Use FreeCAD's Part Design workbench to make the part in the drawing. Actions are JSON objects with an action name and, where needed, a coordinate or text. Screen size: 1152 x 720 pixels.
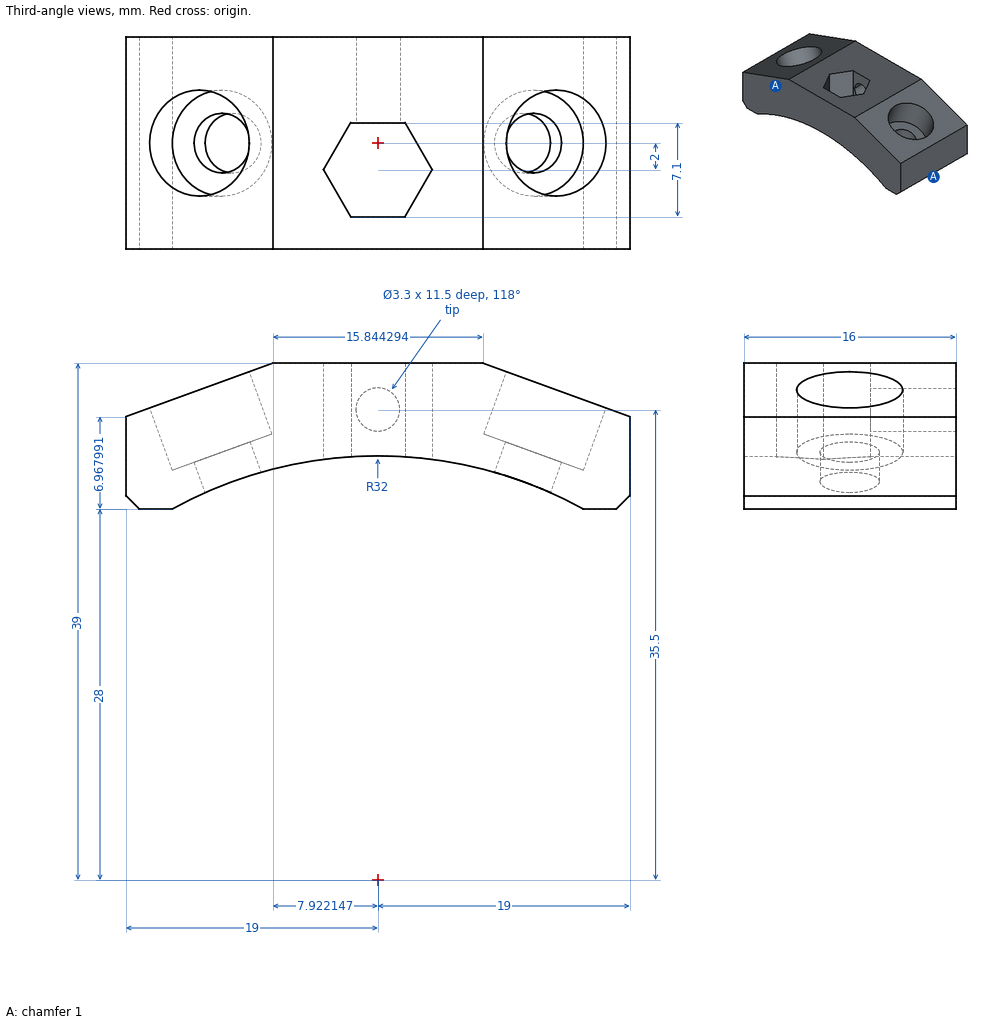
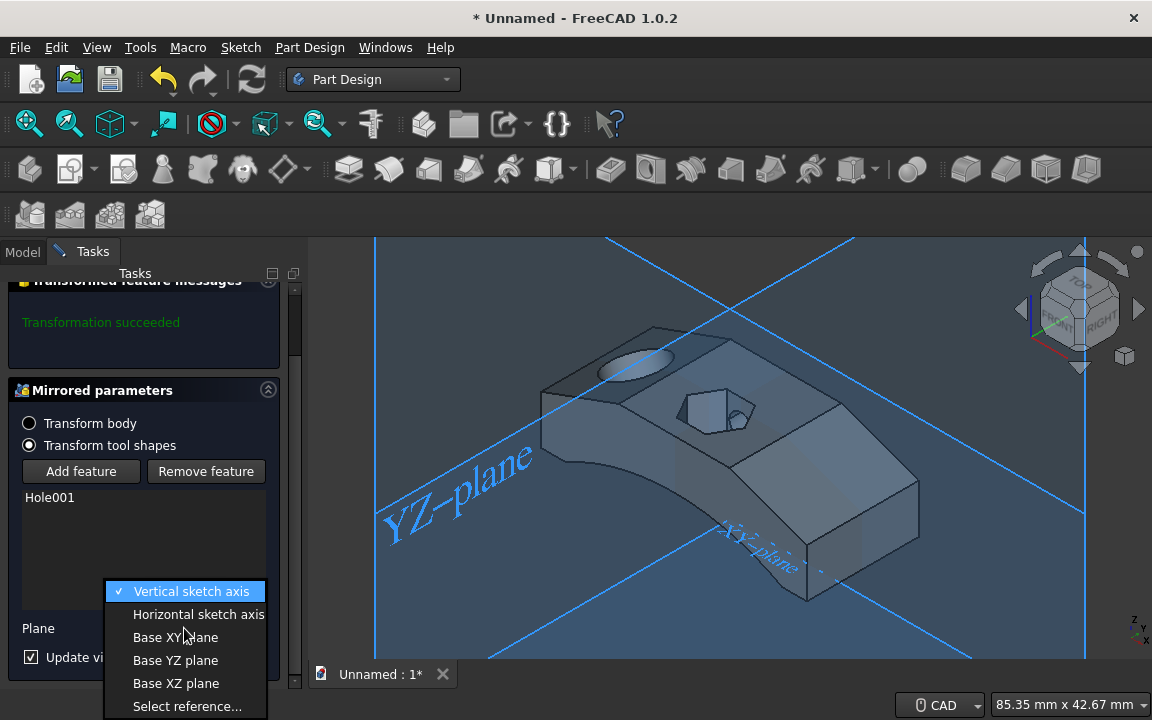
{"action": "left_click", "coordinate": [184, 660]}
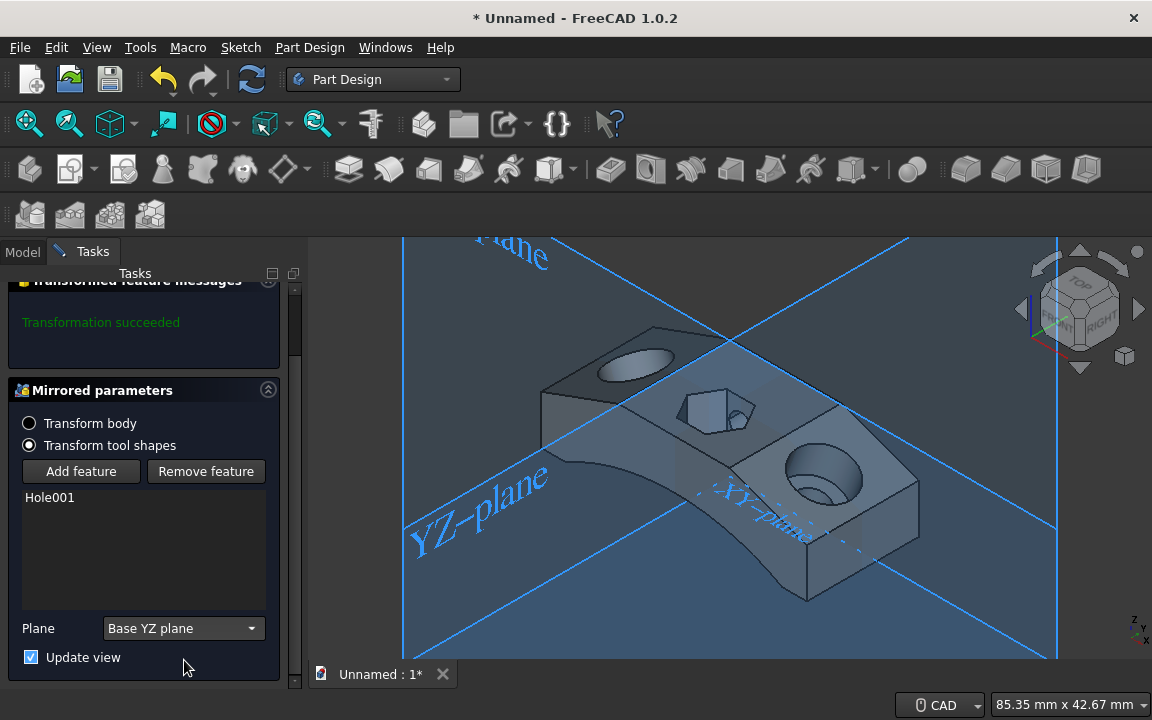
{"action": "scroll", "coordinate": [295, 486], "scroll_direction": "up", "scroll_amount": 2}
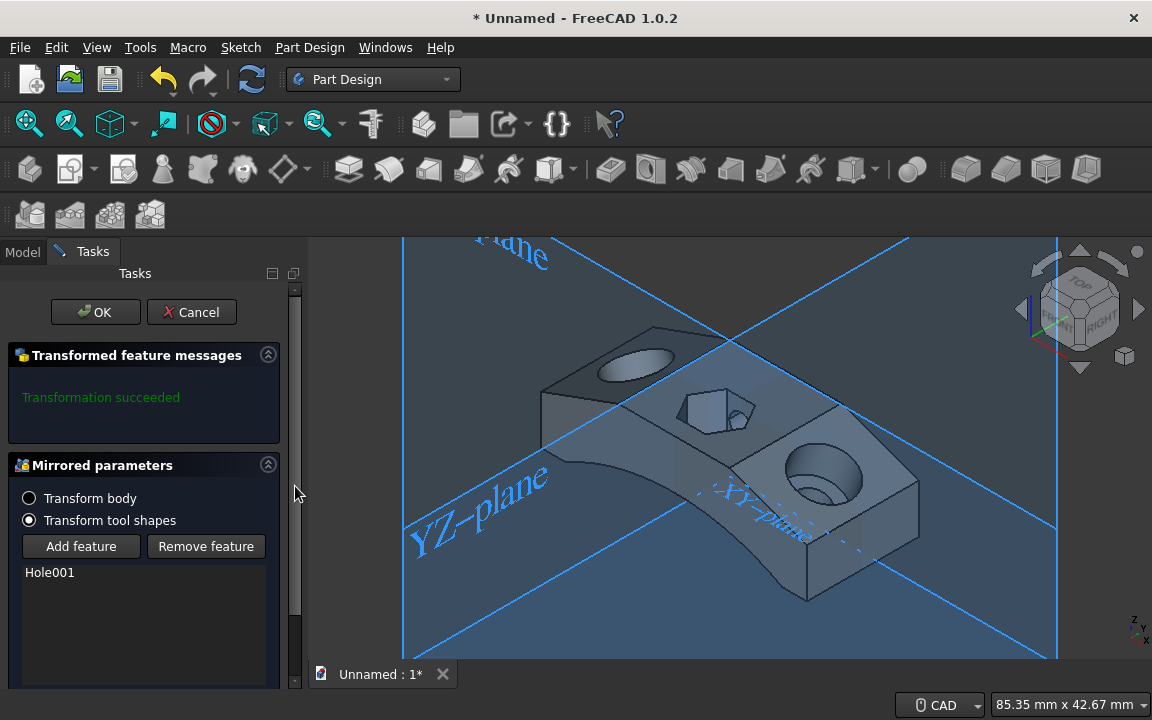
{"action": "left_click", "coordinate": [96, 312]}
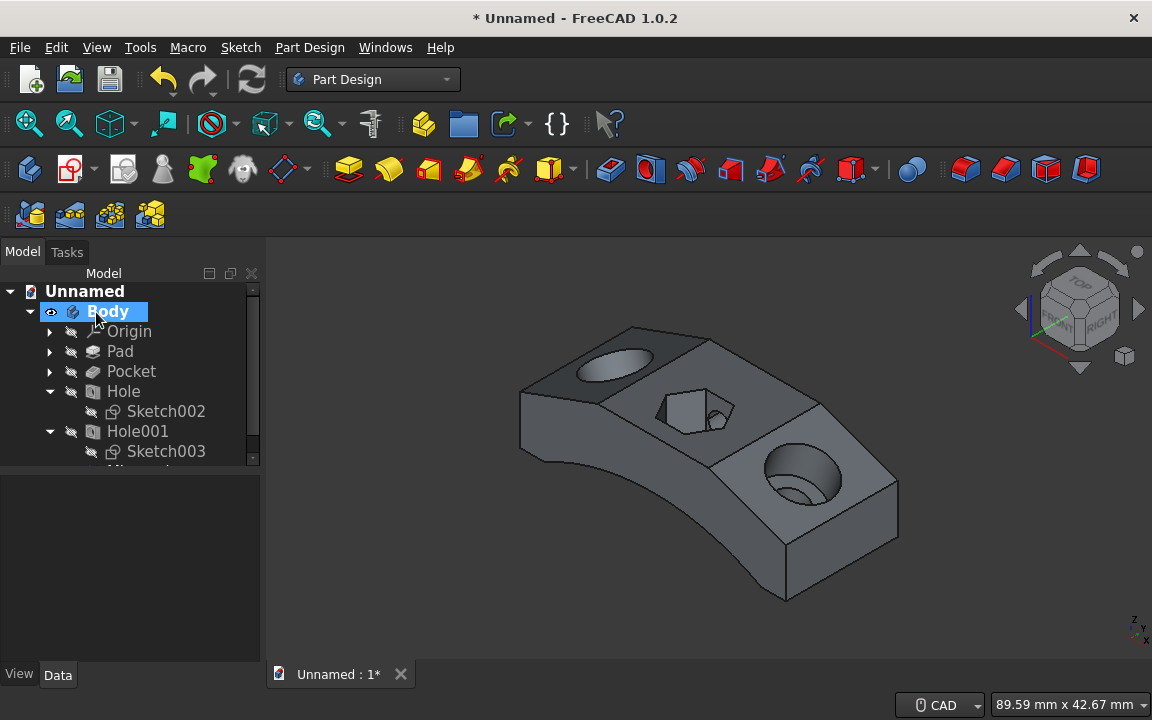
{"action": "key", "text": "2"}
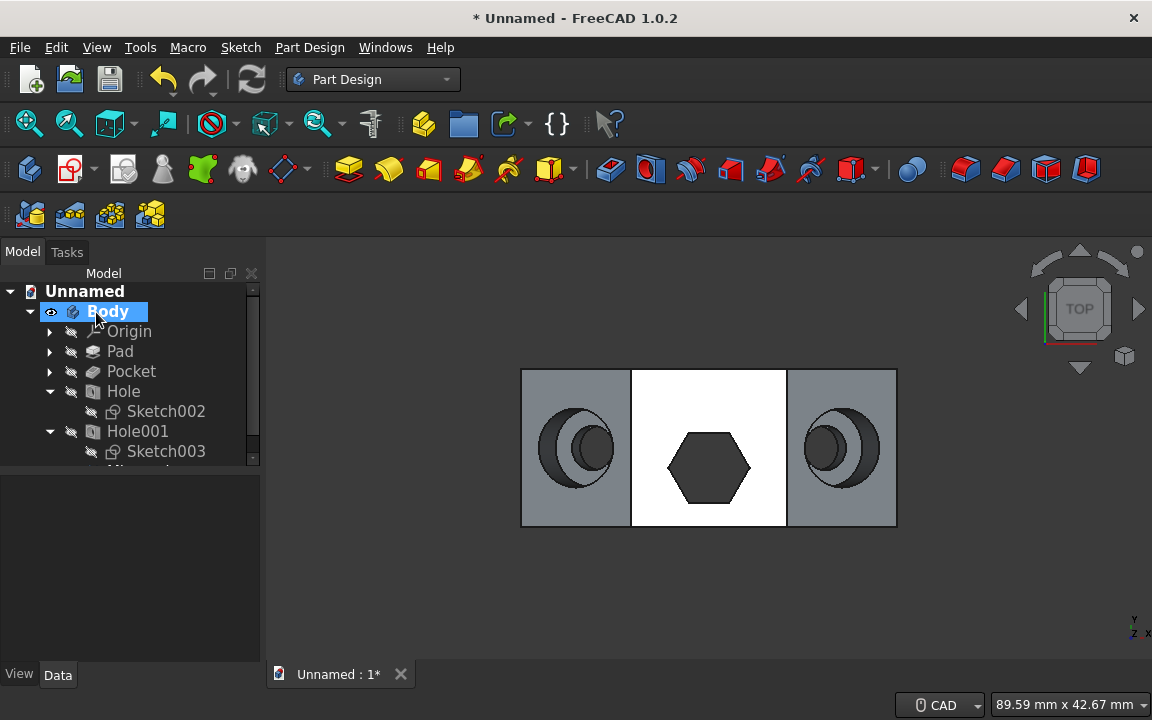
{"action": "key", "text": "v f"}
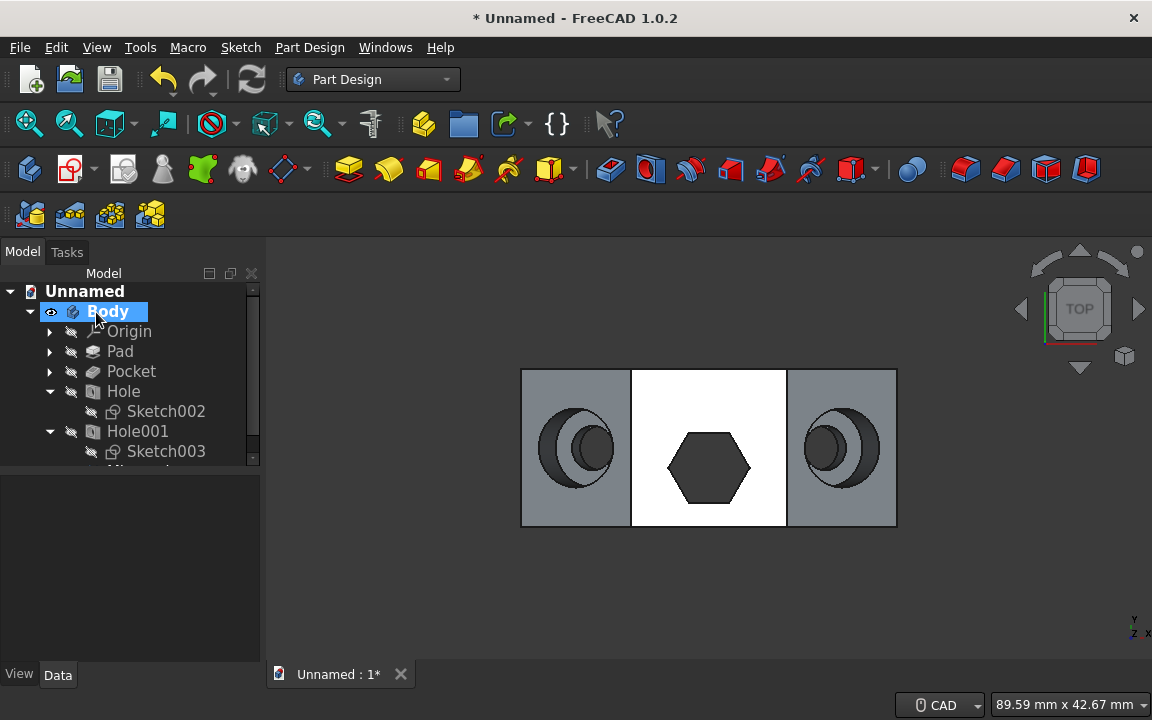
{"action": "key", "text": "0"}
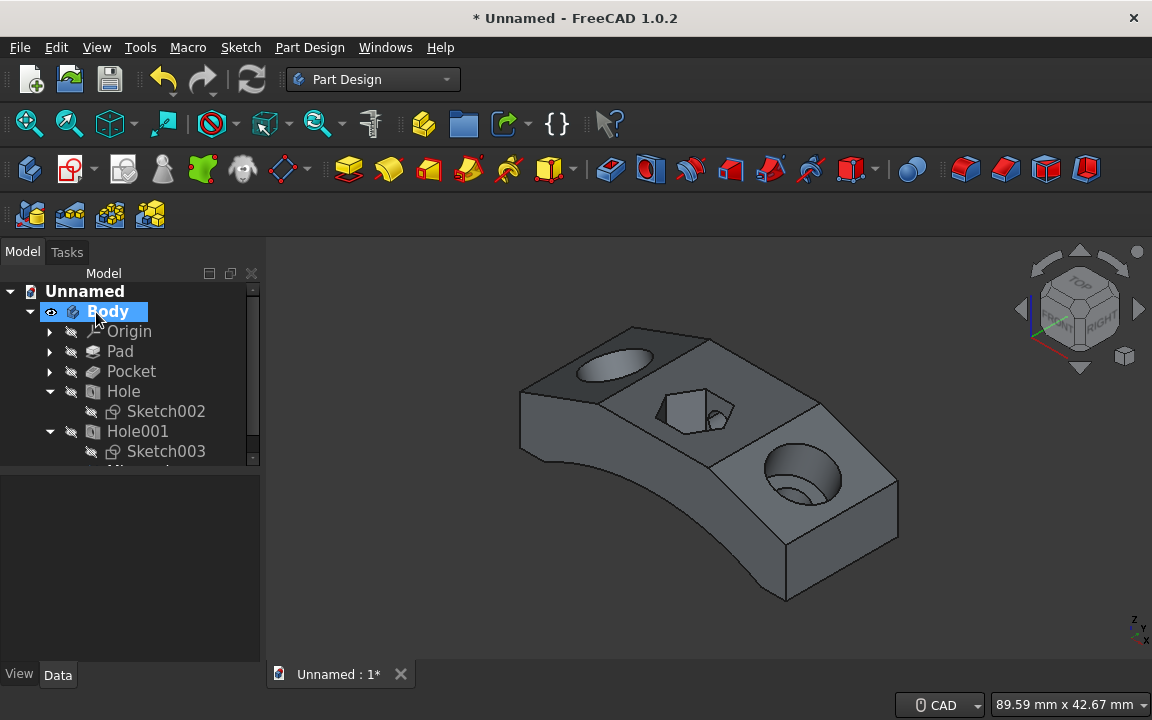
{"action": "key", "text": "1"}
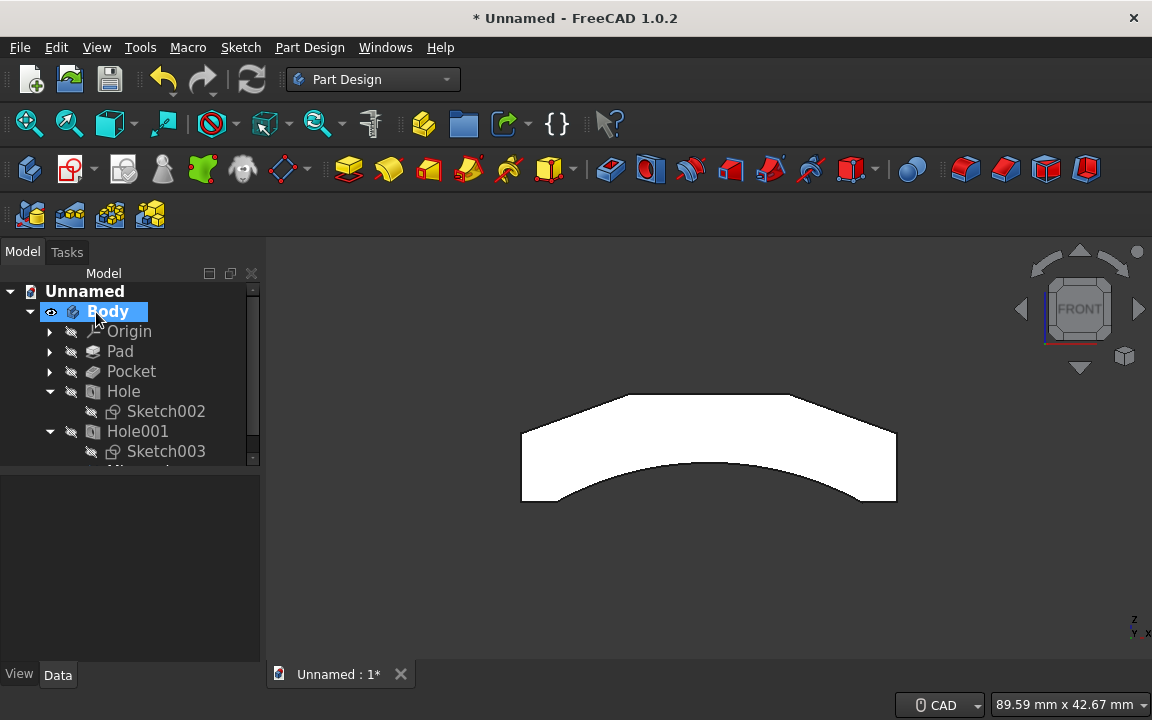
{"action": "key", "text": "v f"}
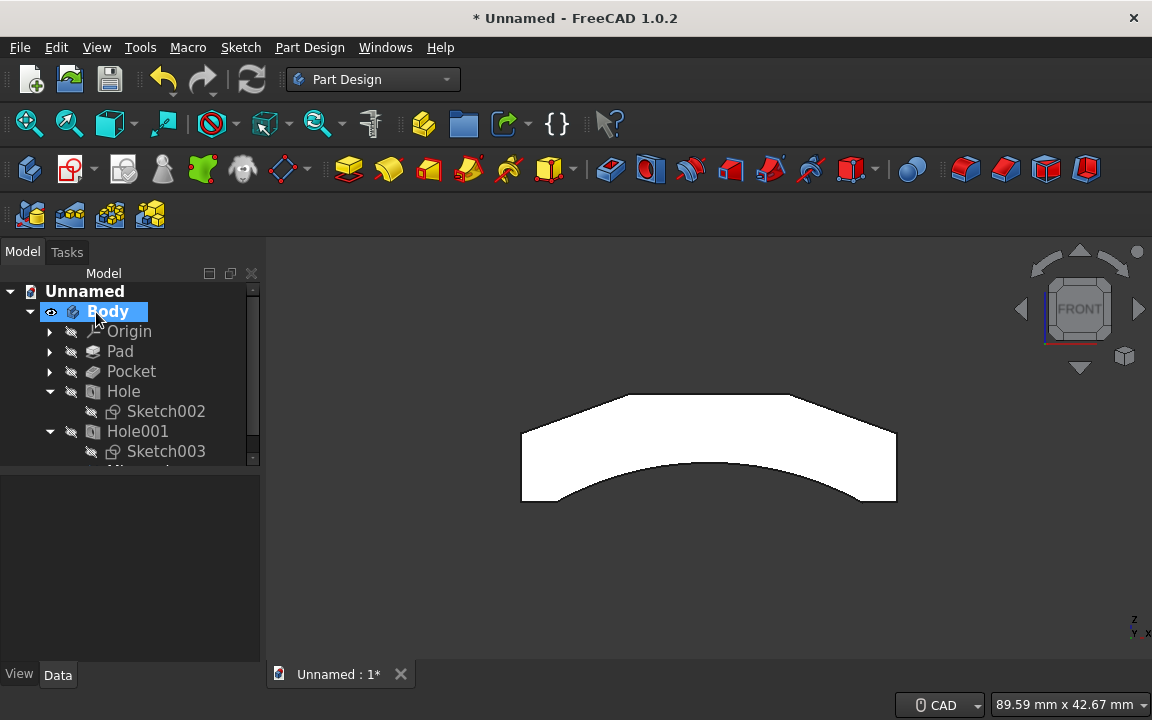
{"action": "key", "text": "3"}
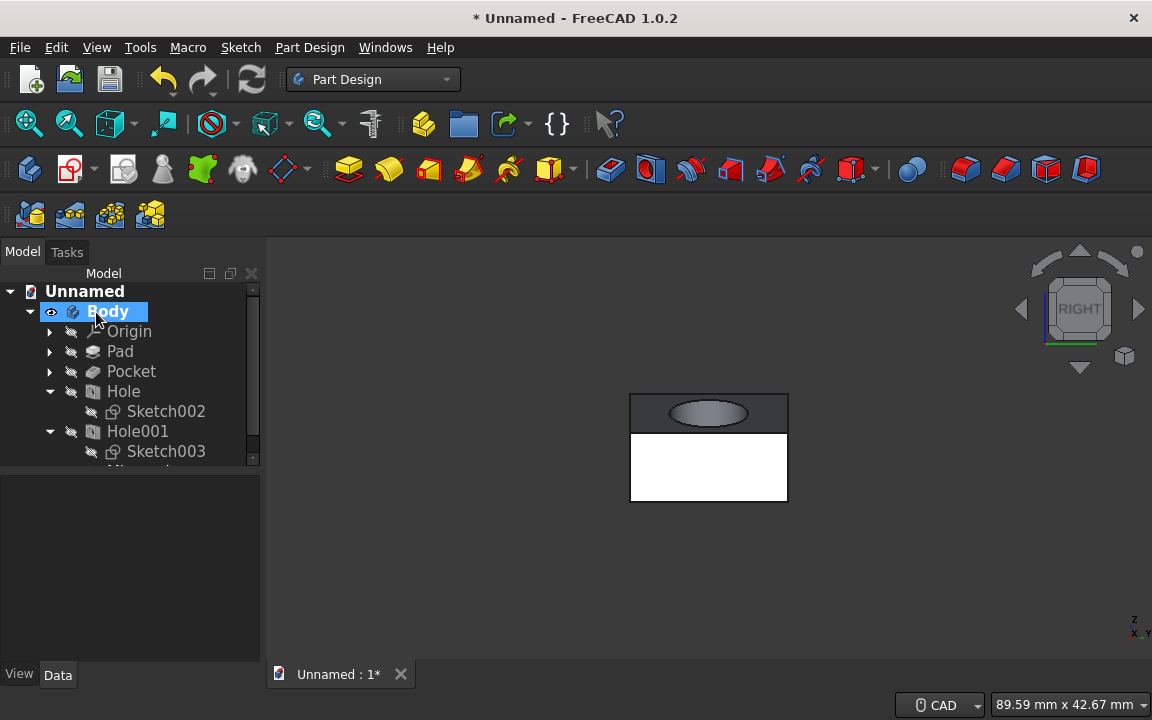
{"action": "key", "text": "v f"}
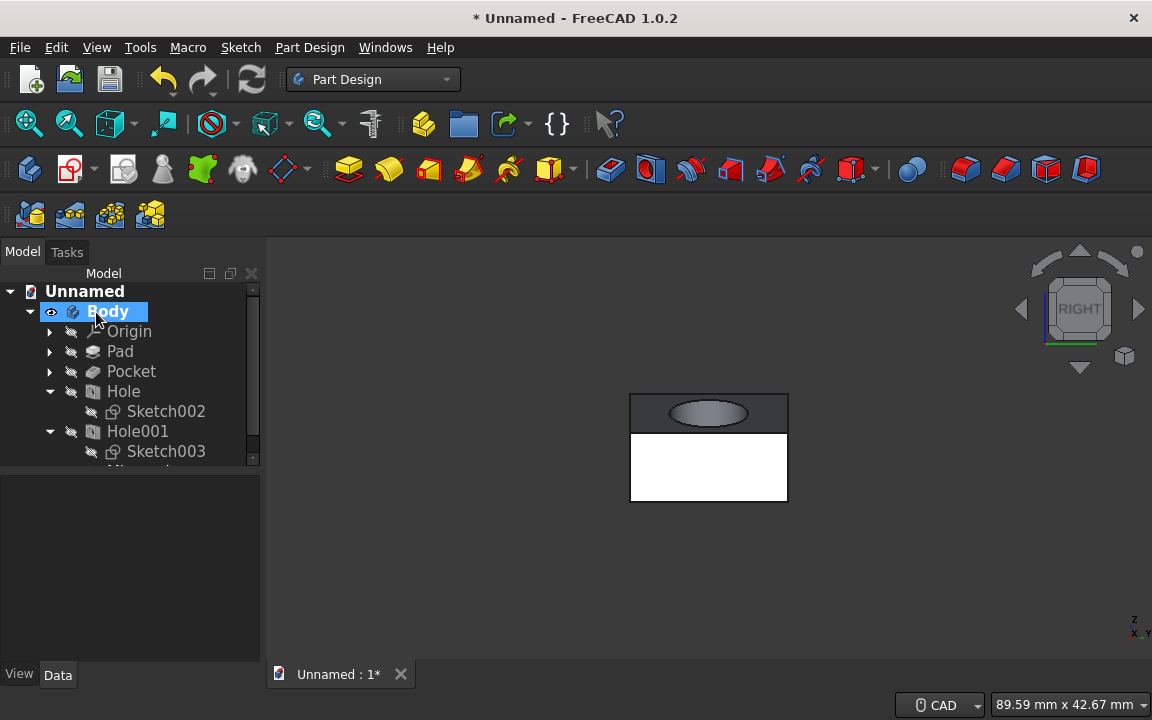
{"action": "left_click", "coordinate": [709, 501]}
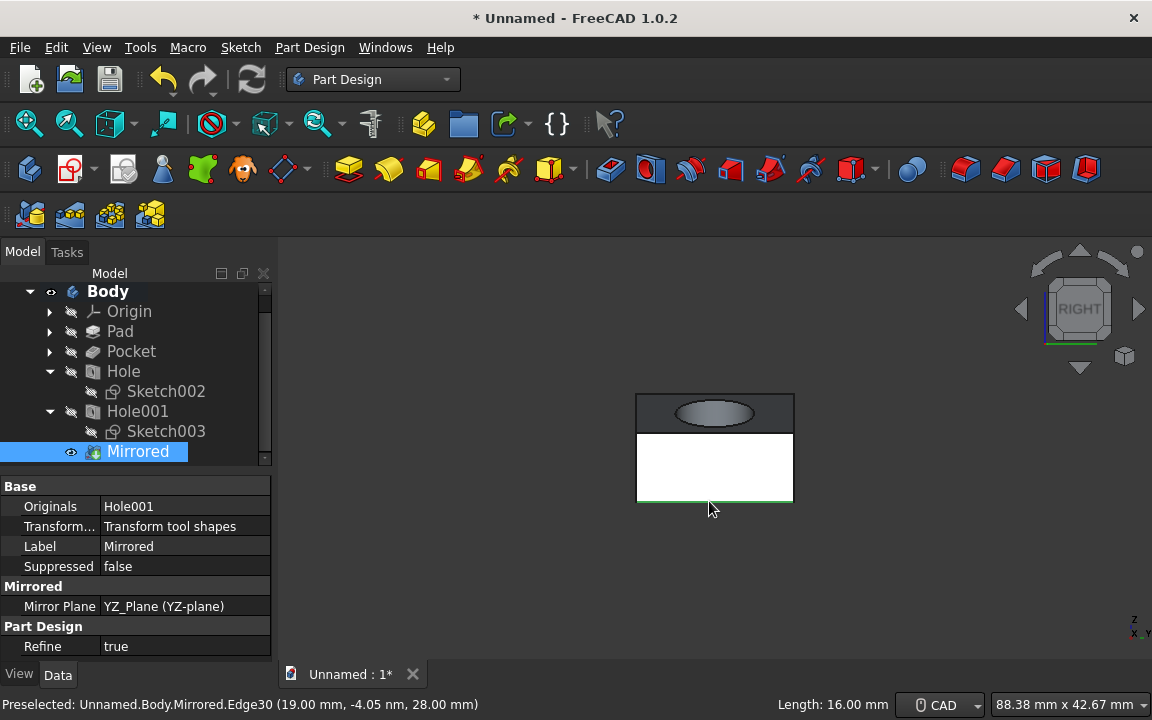
{"action": "key", "text": "5"}